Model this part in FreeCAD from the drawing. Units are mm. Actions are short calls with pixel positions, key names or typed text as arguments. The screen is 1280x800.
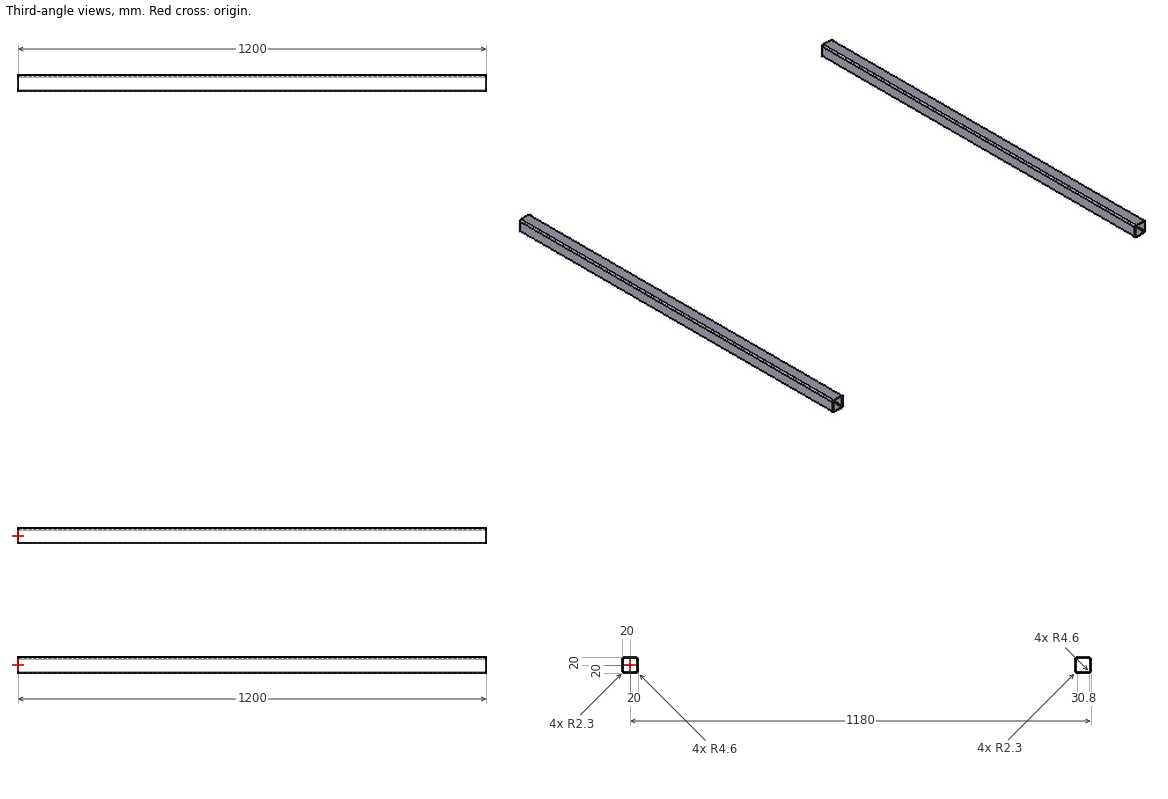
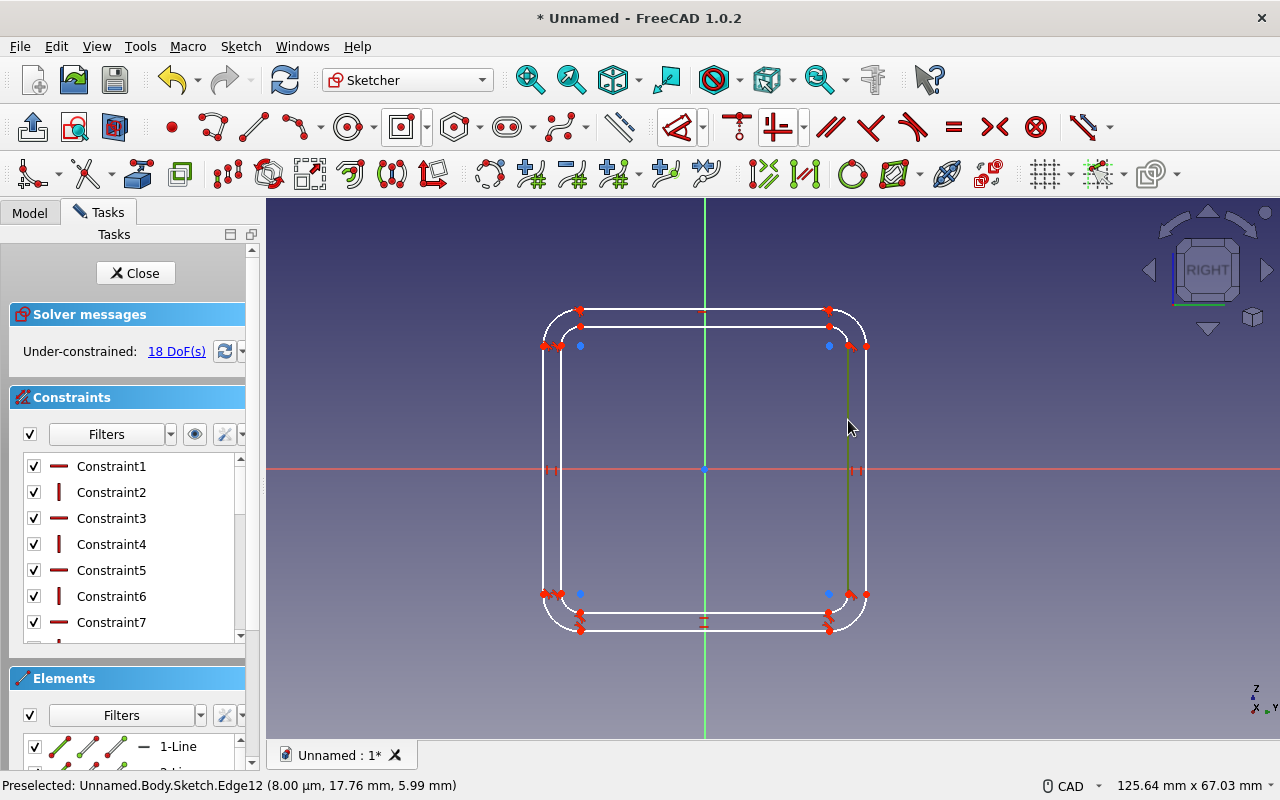
click(842, 332)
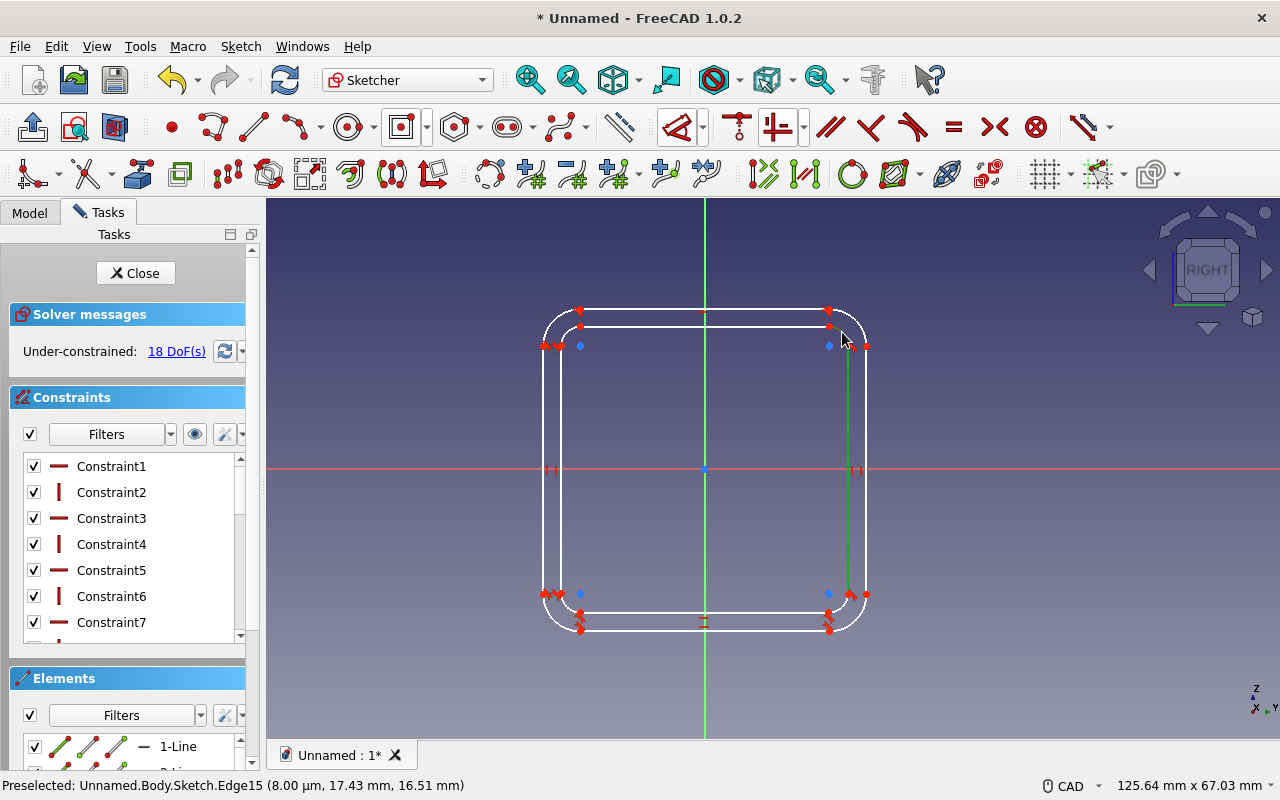
key(t)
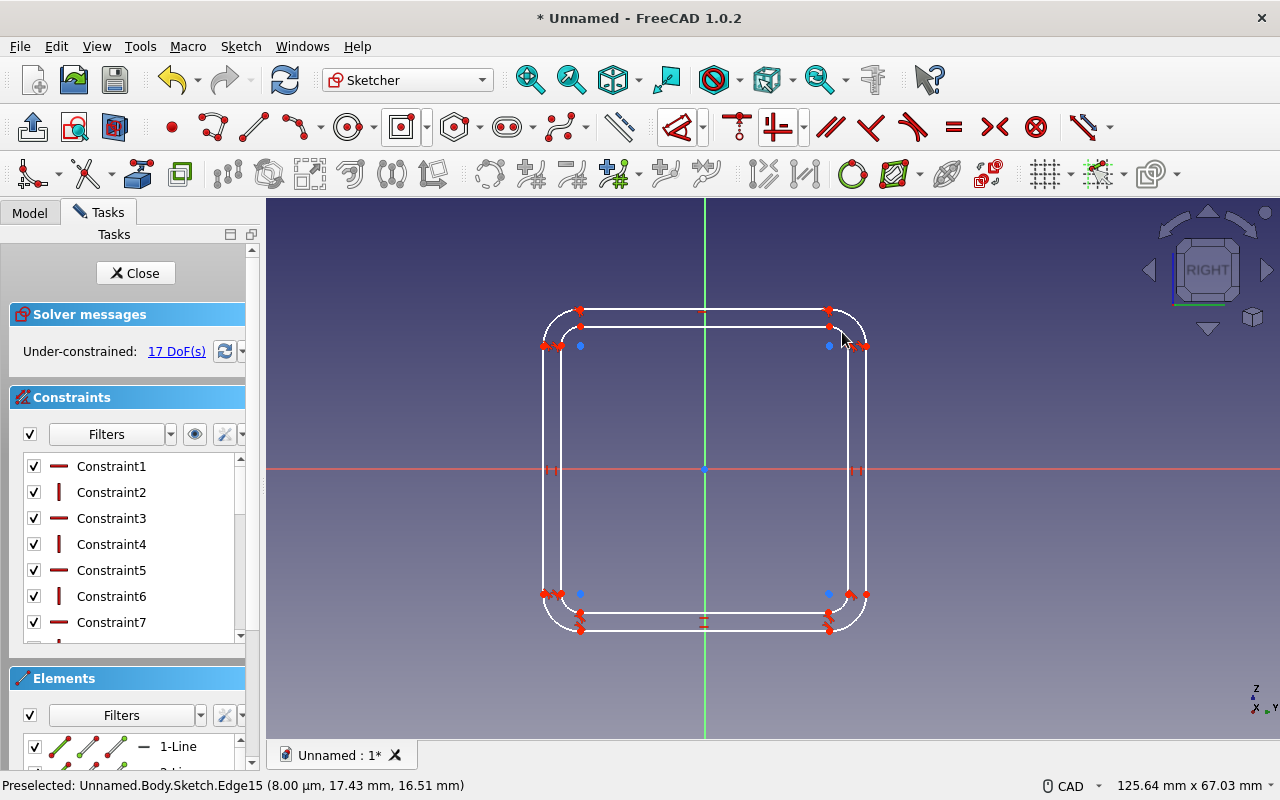
click(848, 420)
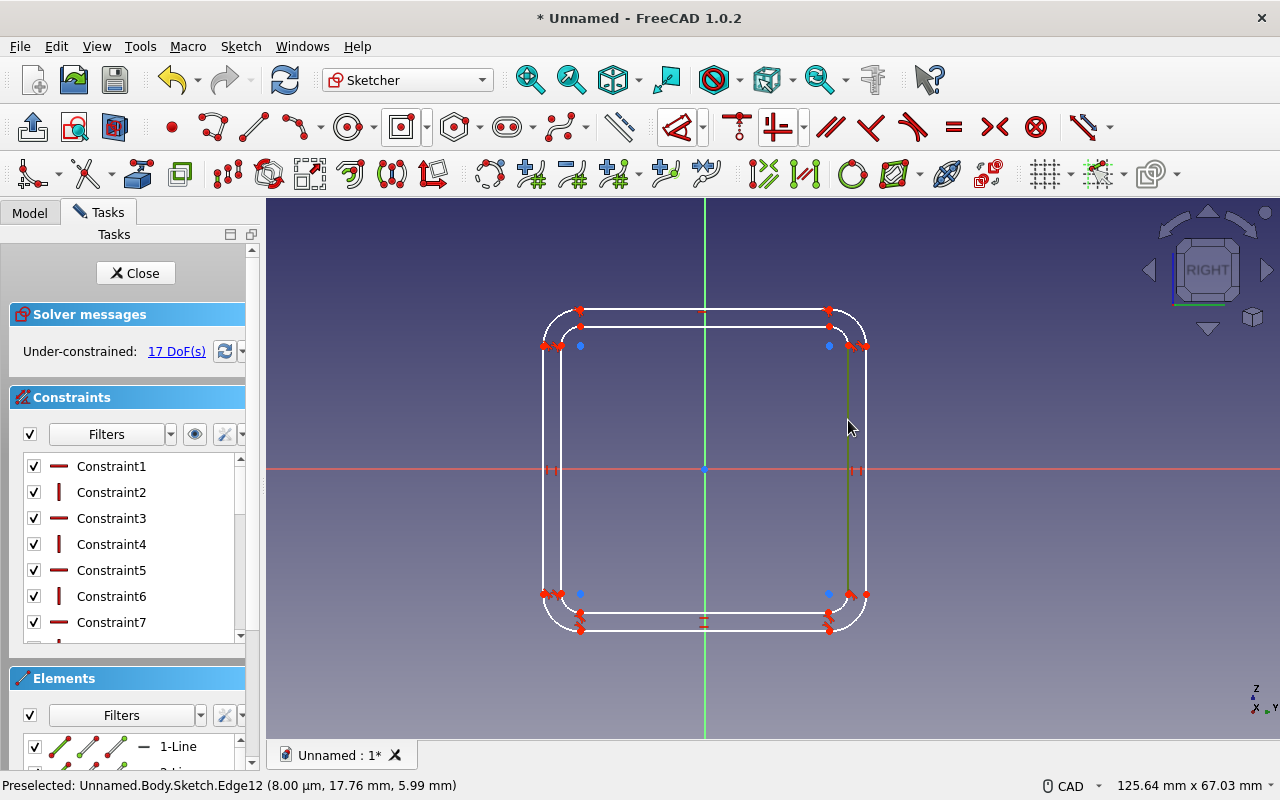
click(842, 607)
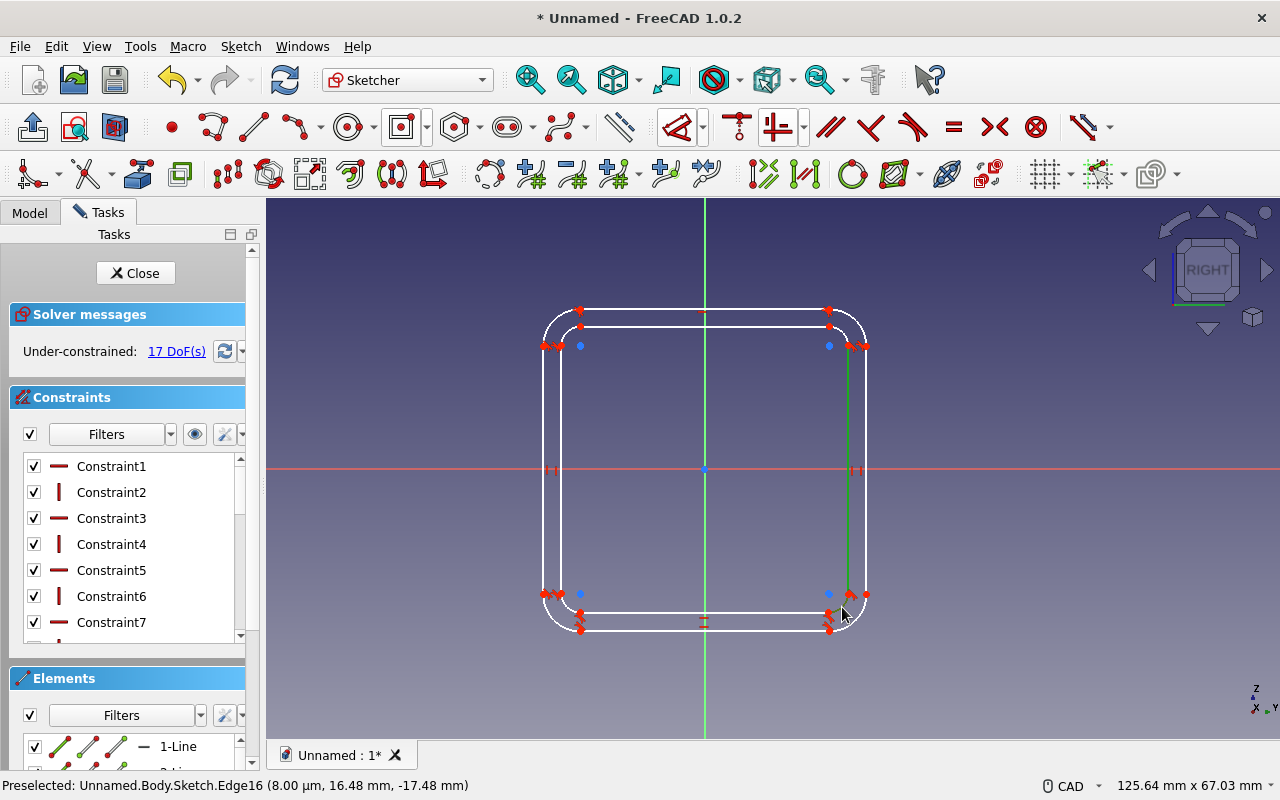
click(913, 128)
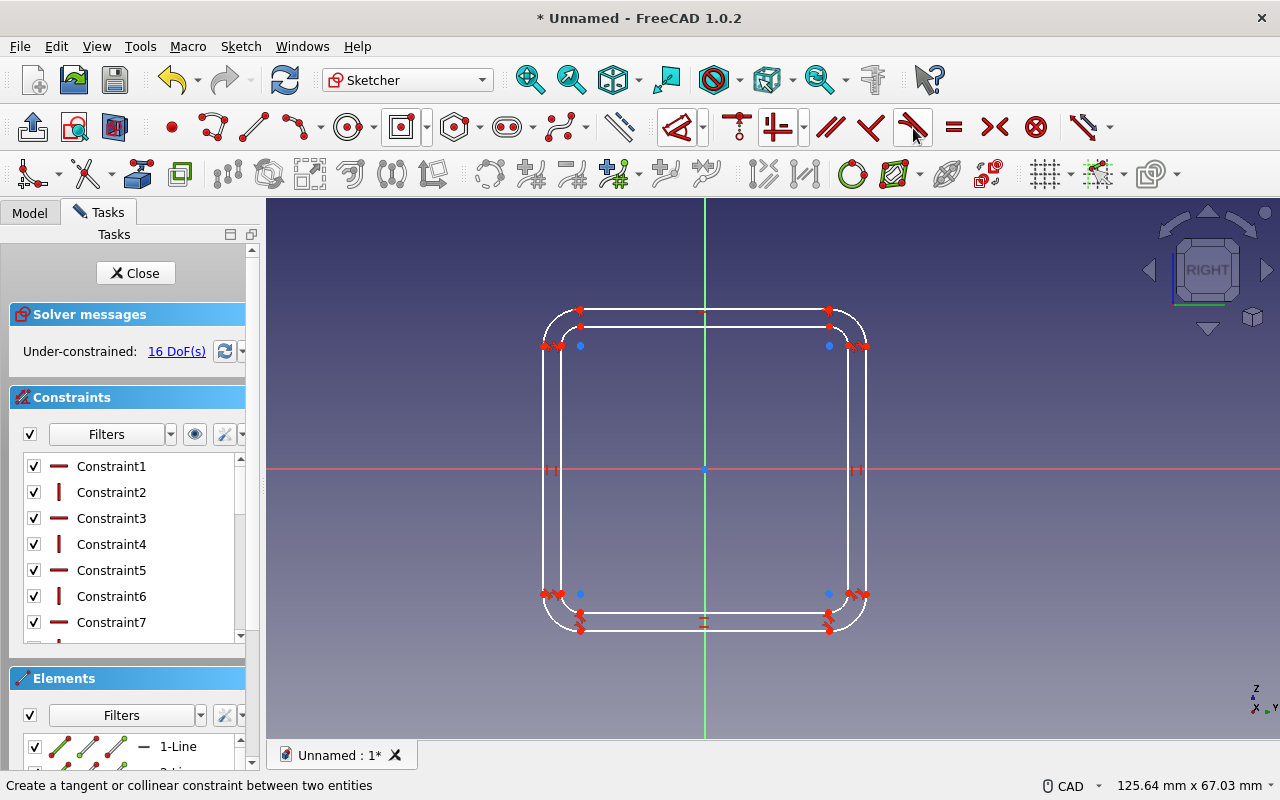
click(547, 611)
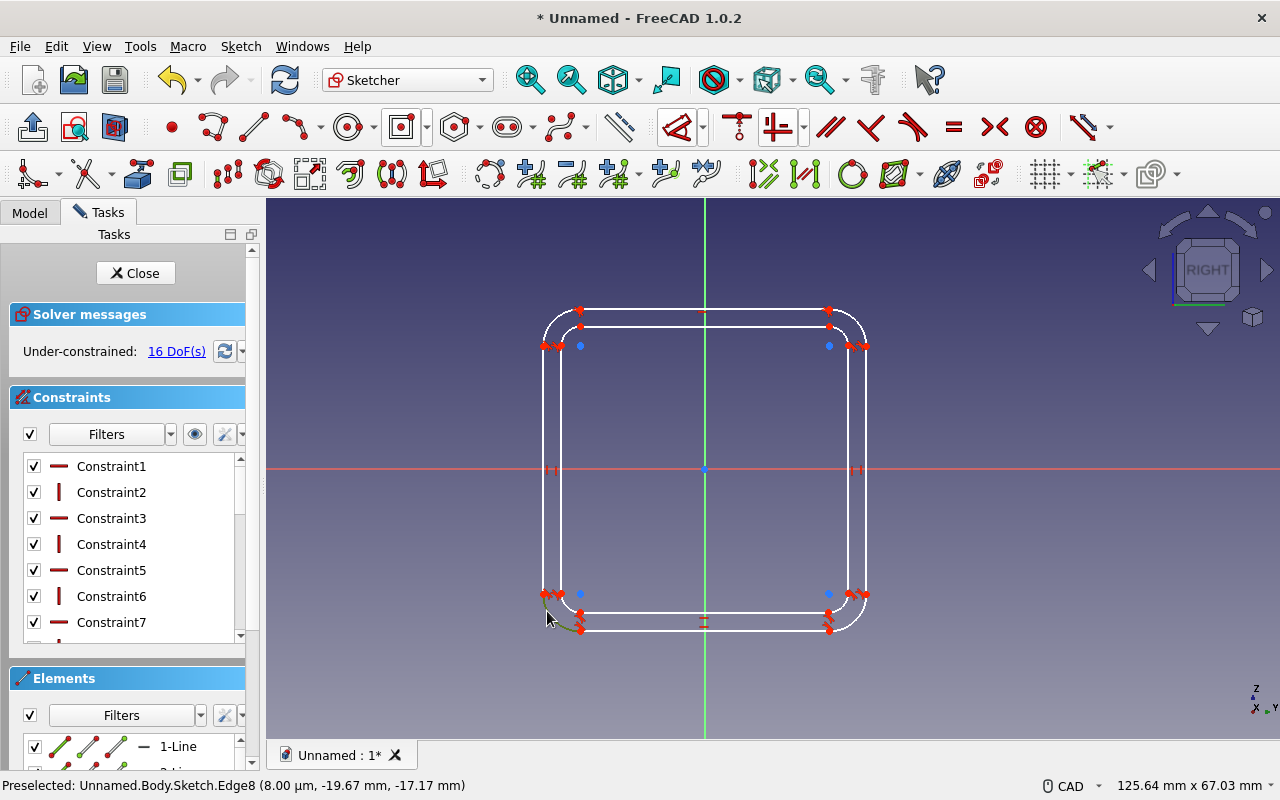
click(567, 607)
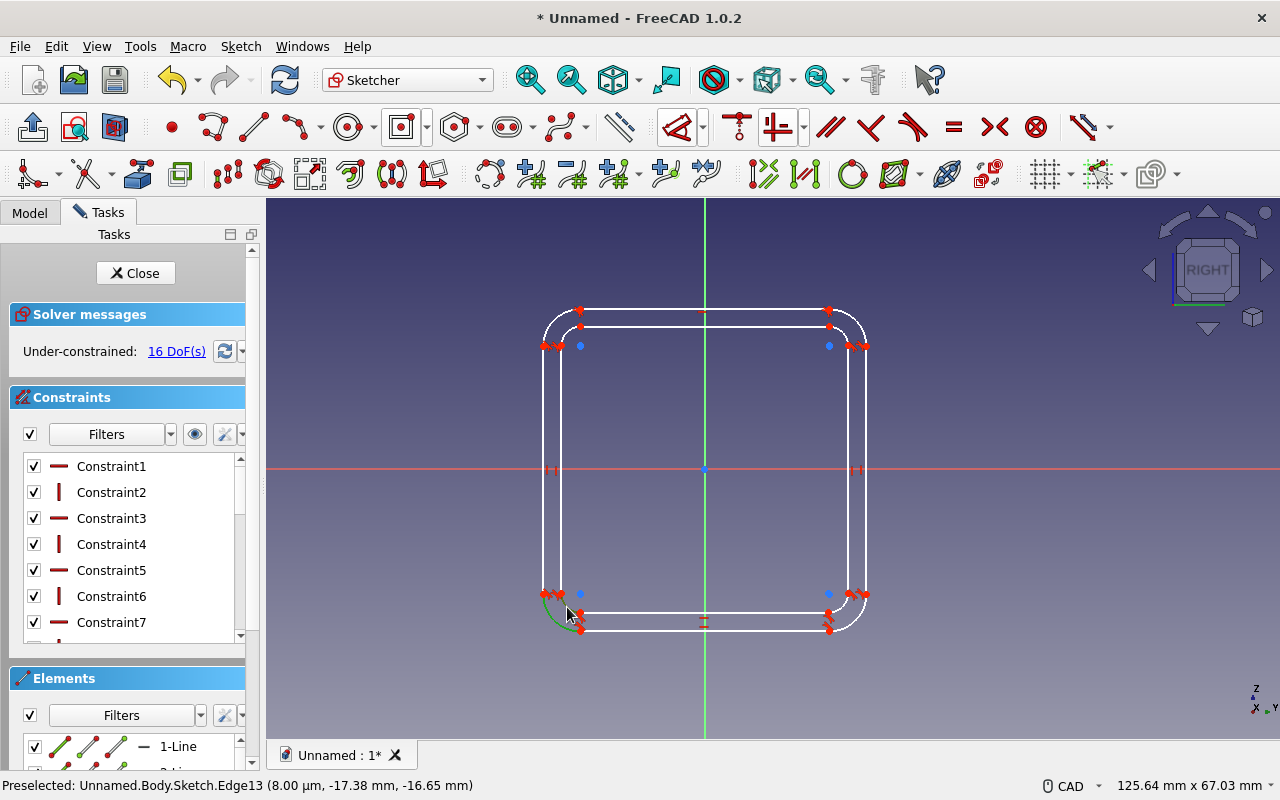
key(c)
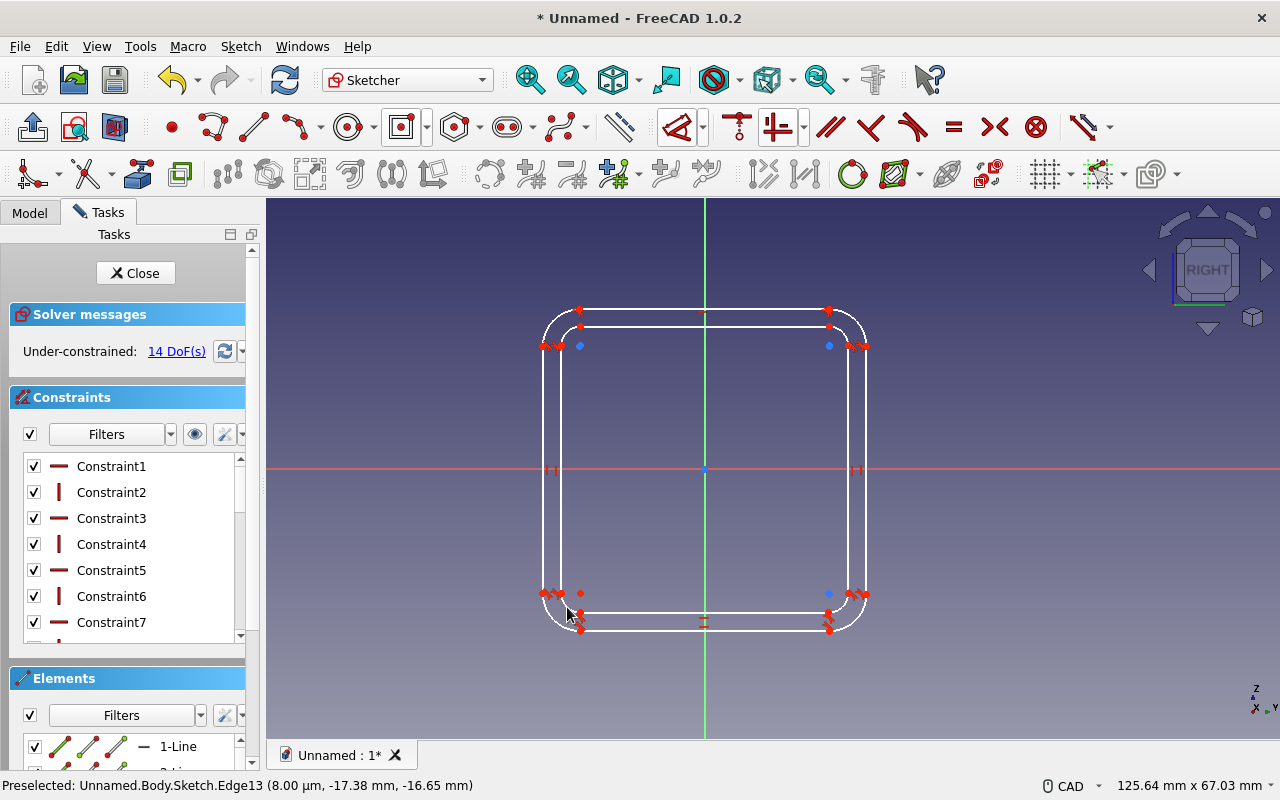
click(563, 313)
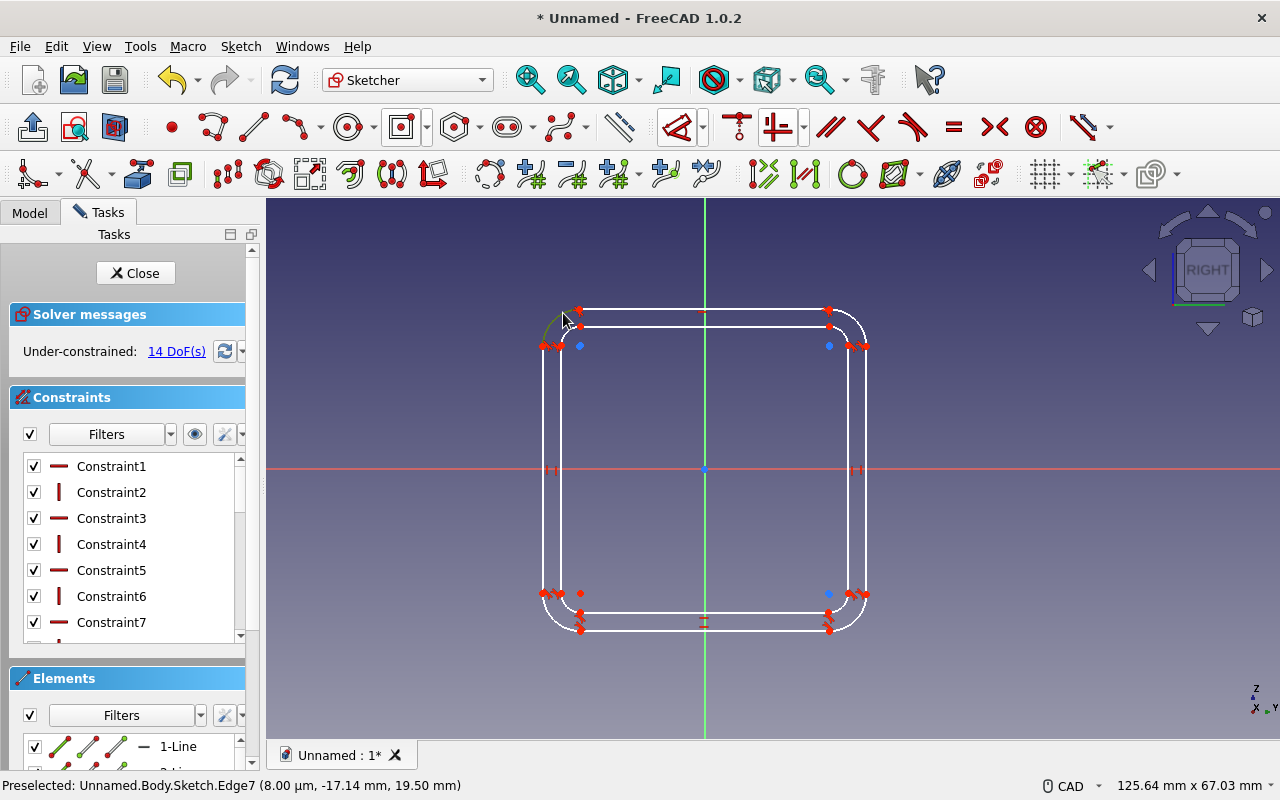
click(567, 332)